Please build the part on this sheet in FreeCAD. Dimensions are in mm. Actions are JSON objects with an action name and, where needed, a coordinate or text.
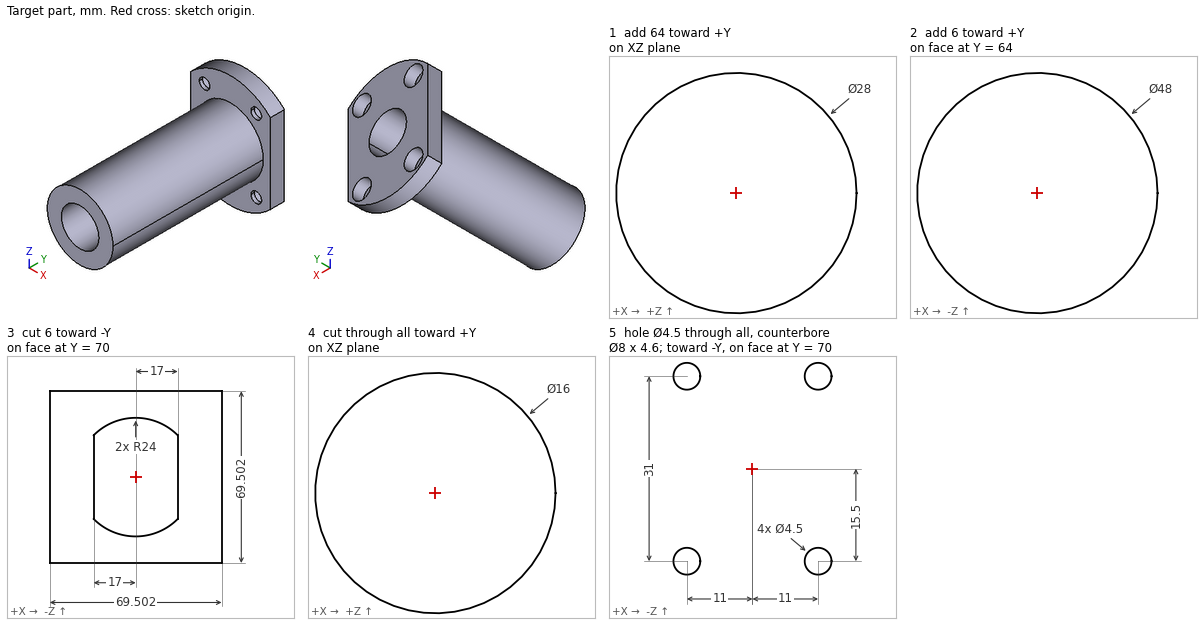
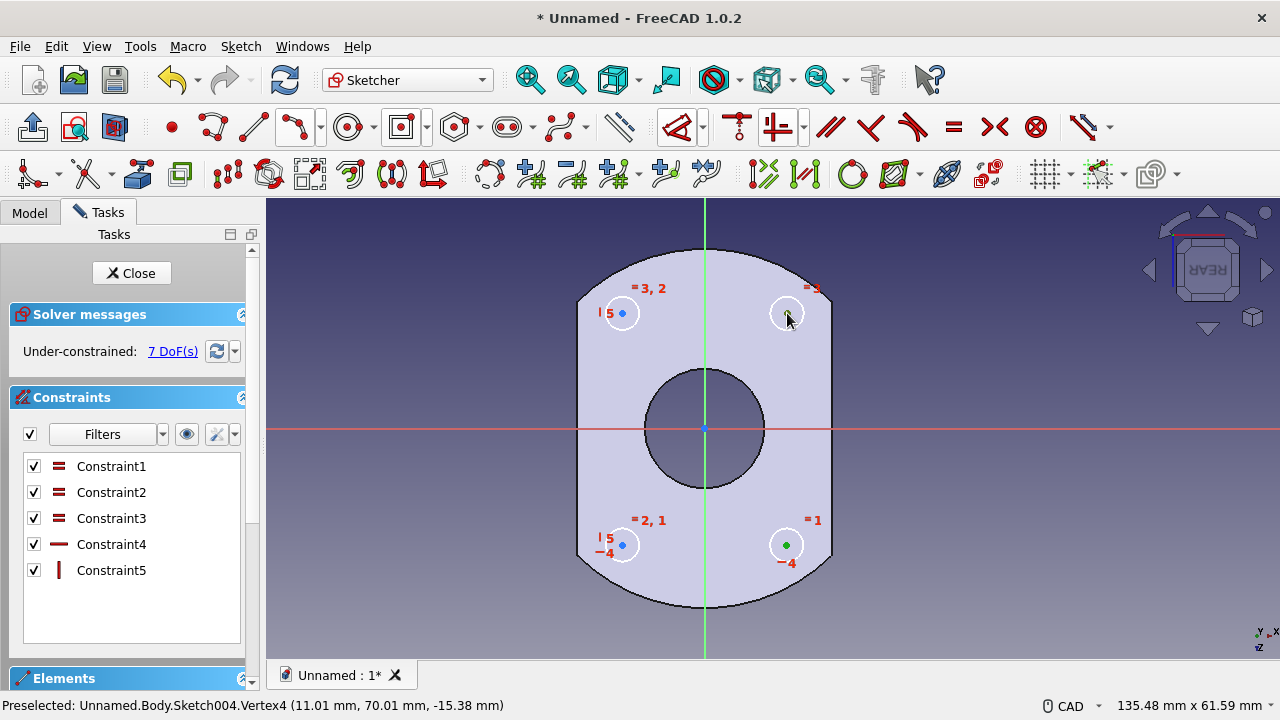
{"action": "key", "text": "v"}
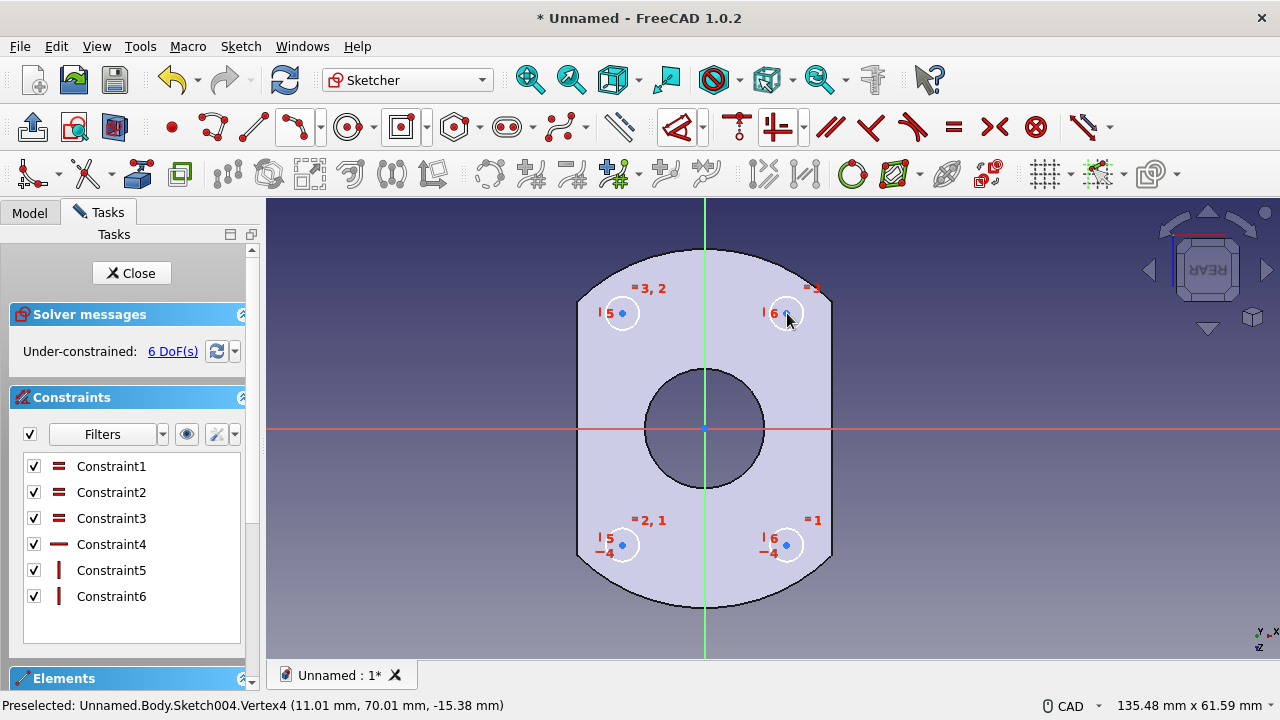
{"action": "left_click", "coordinate": [622, 313]}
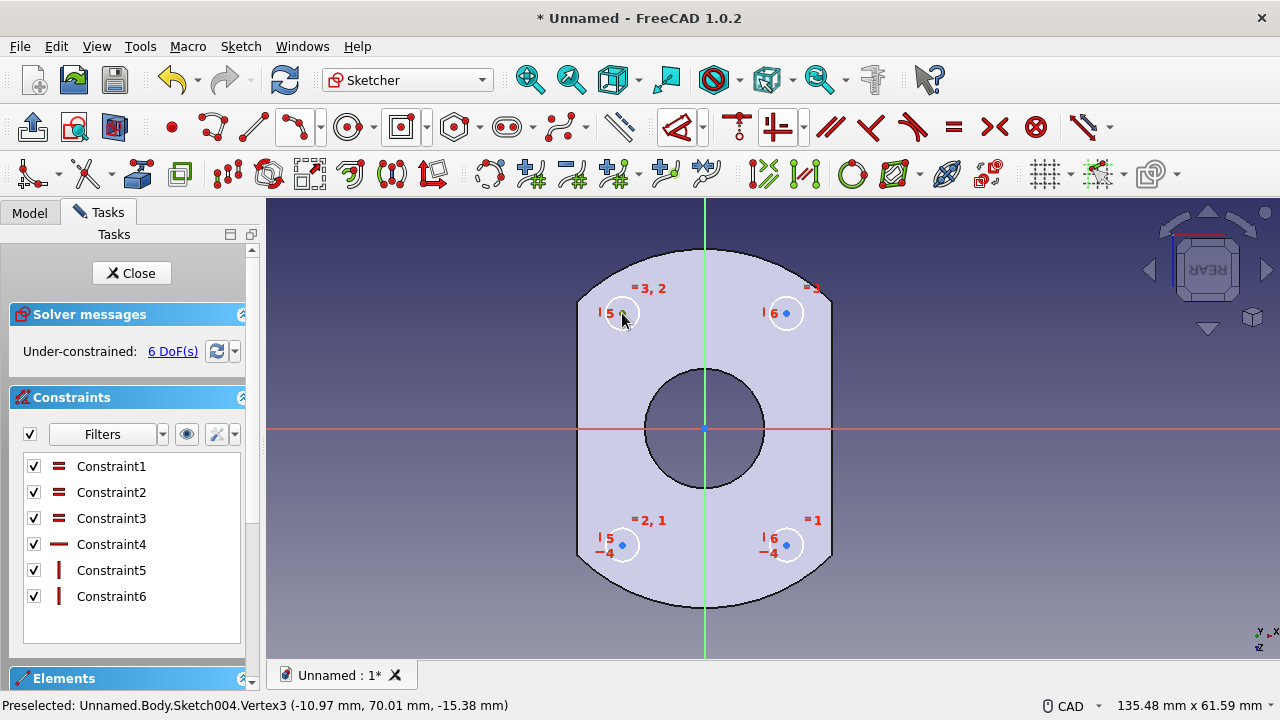
{"action": "left_click", "coordinate": [787, 313]}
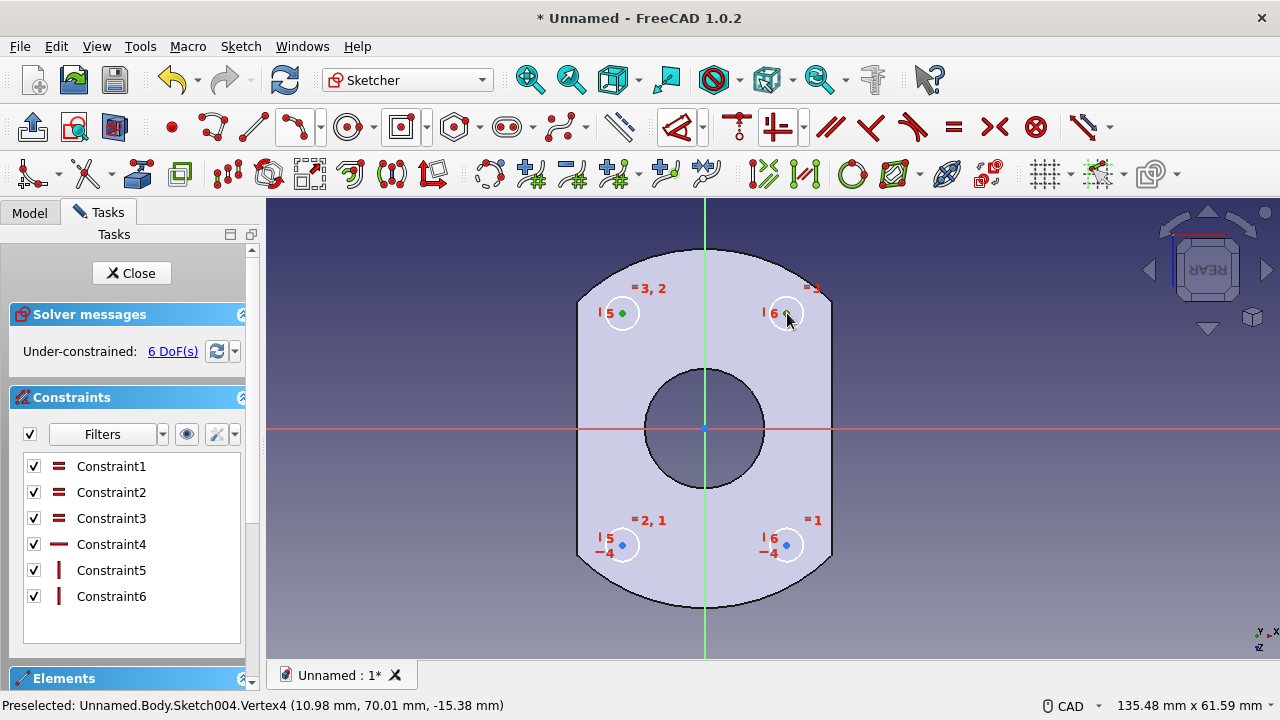
{"action": "left_click", "coordinate": [804, 128]}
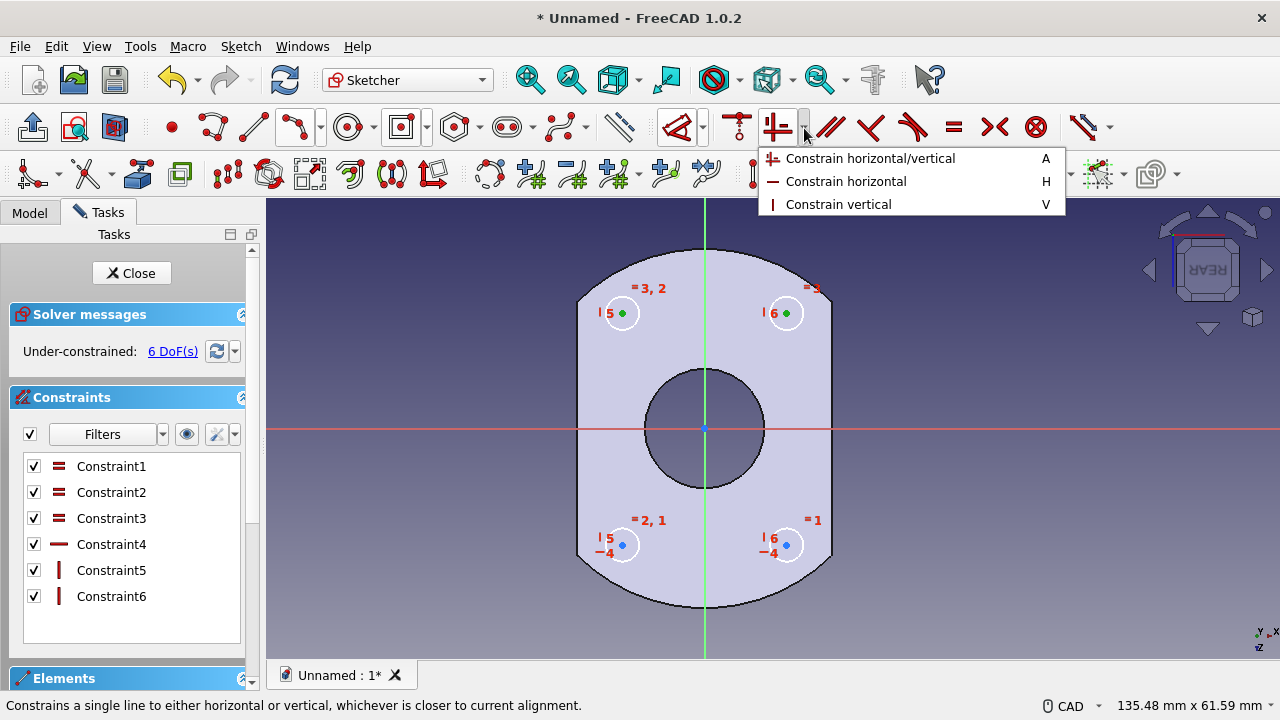
{"action": "left_click", "coordinate": [912, 182]}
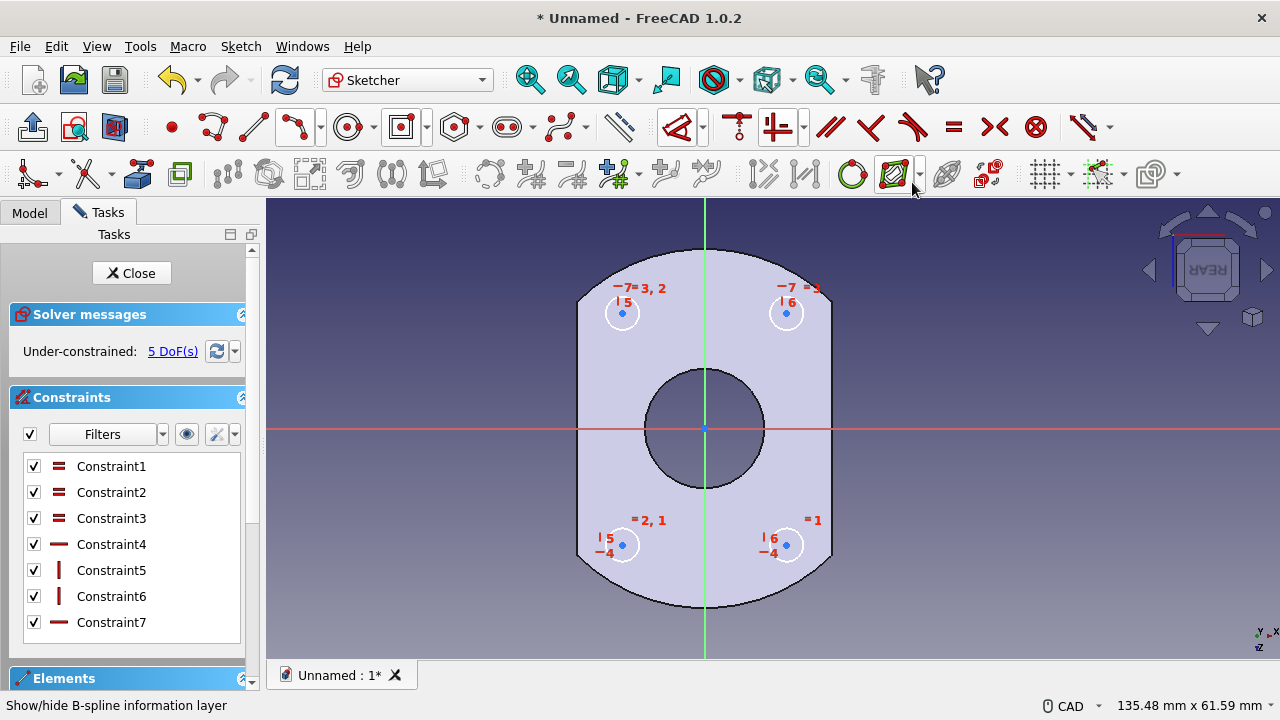
{"action": "left_click", "coordinate": [798, 533]}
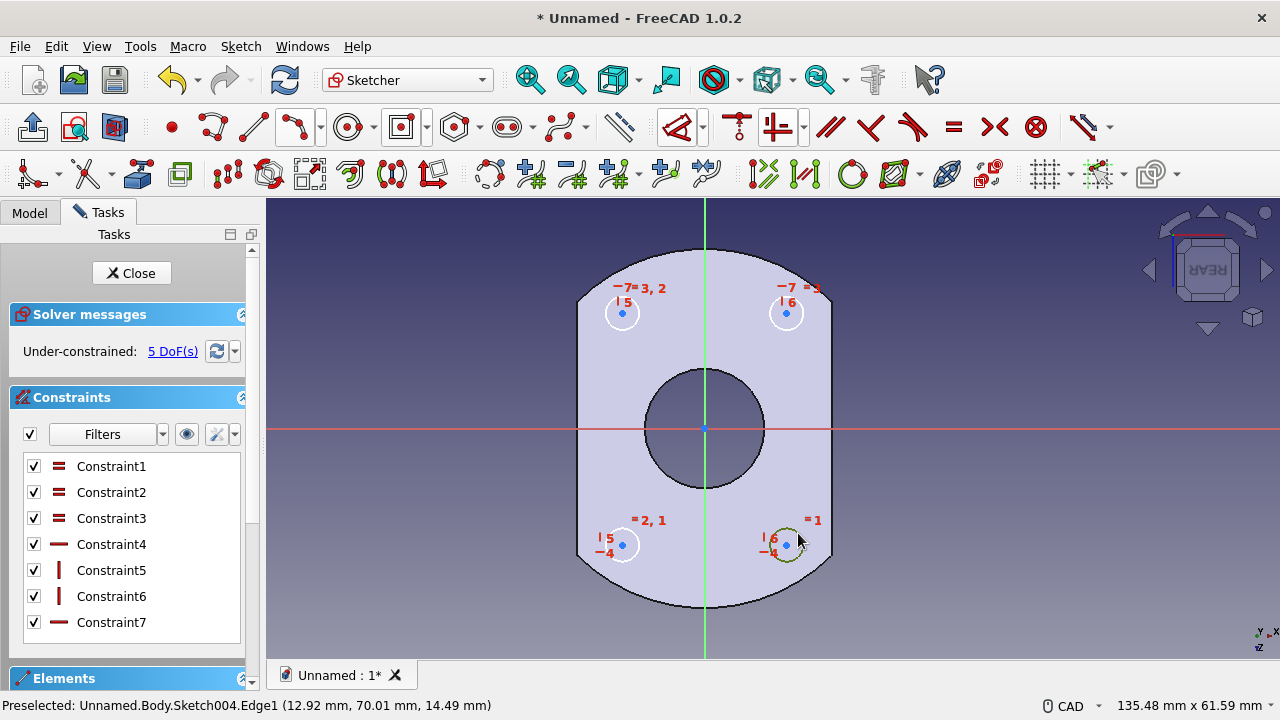
{"action": "left_click", "coordinate": [702, 128]}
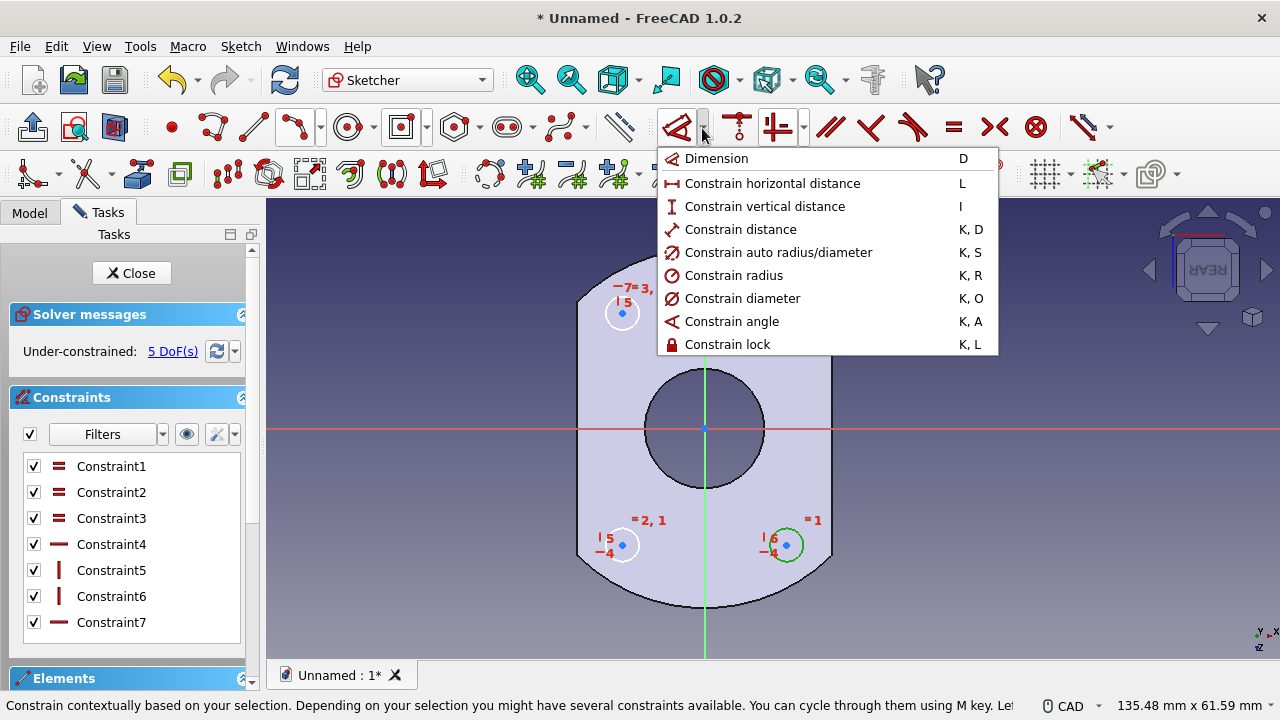
{"action": "left_click", "coordinate": [828, 298]}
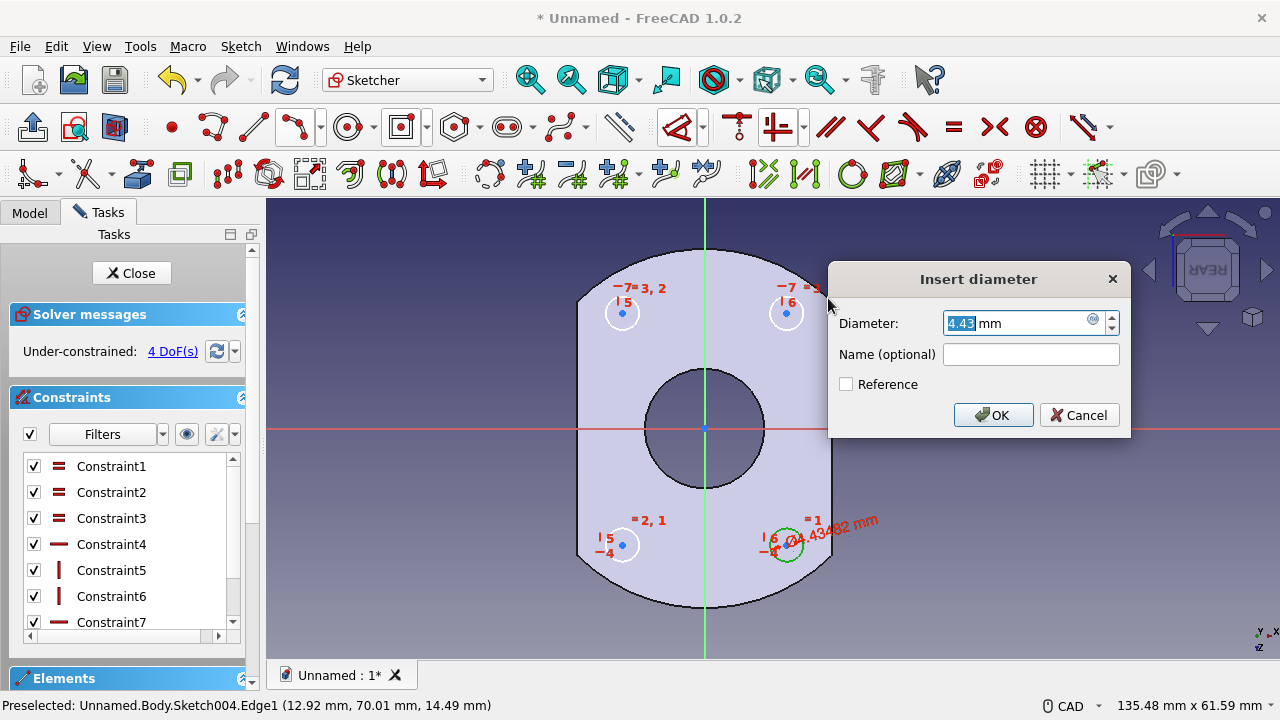
{"action": "type", "text": "4.5"}
{"action": "key", "text": "Return"}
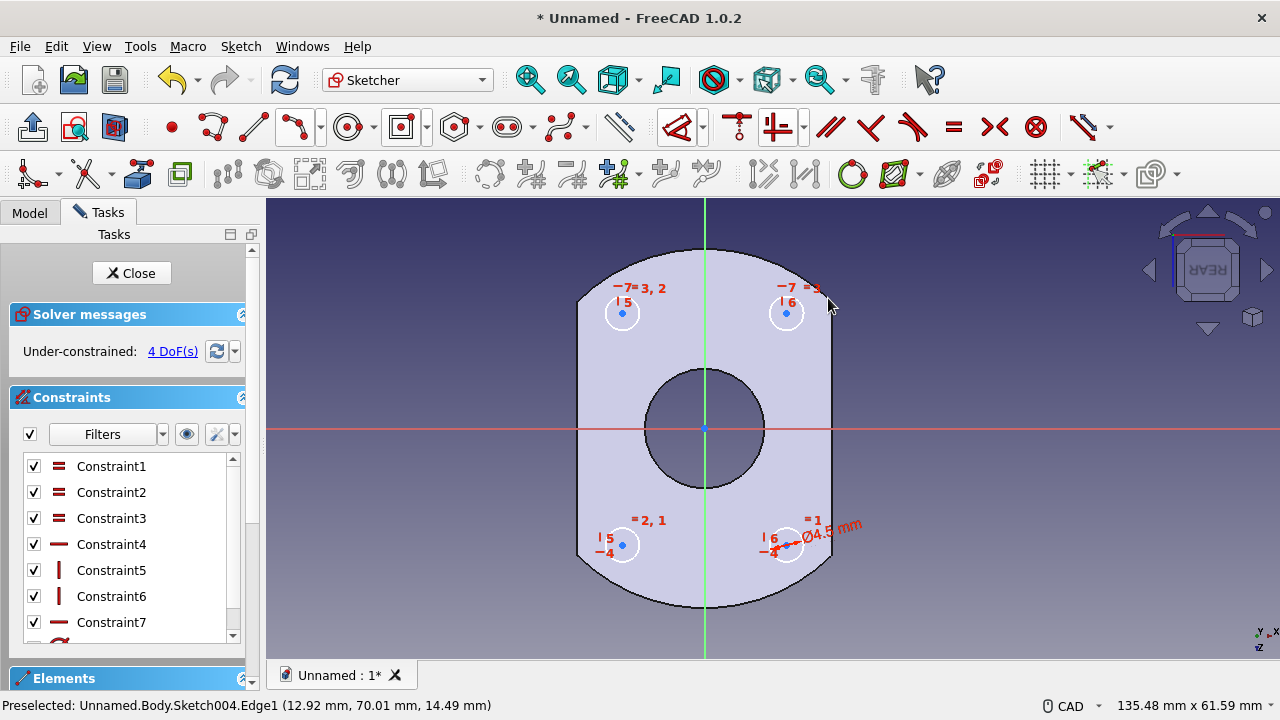
{"action": "left_click", "coordinate": [787, 545]}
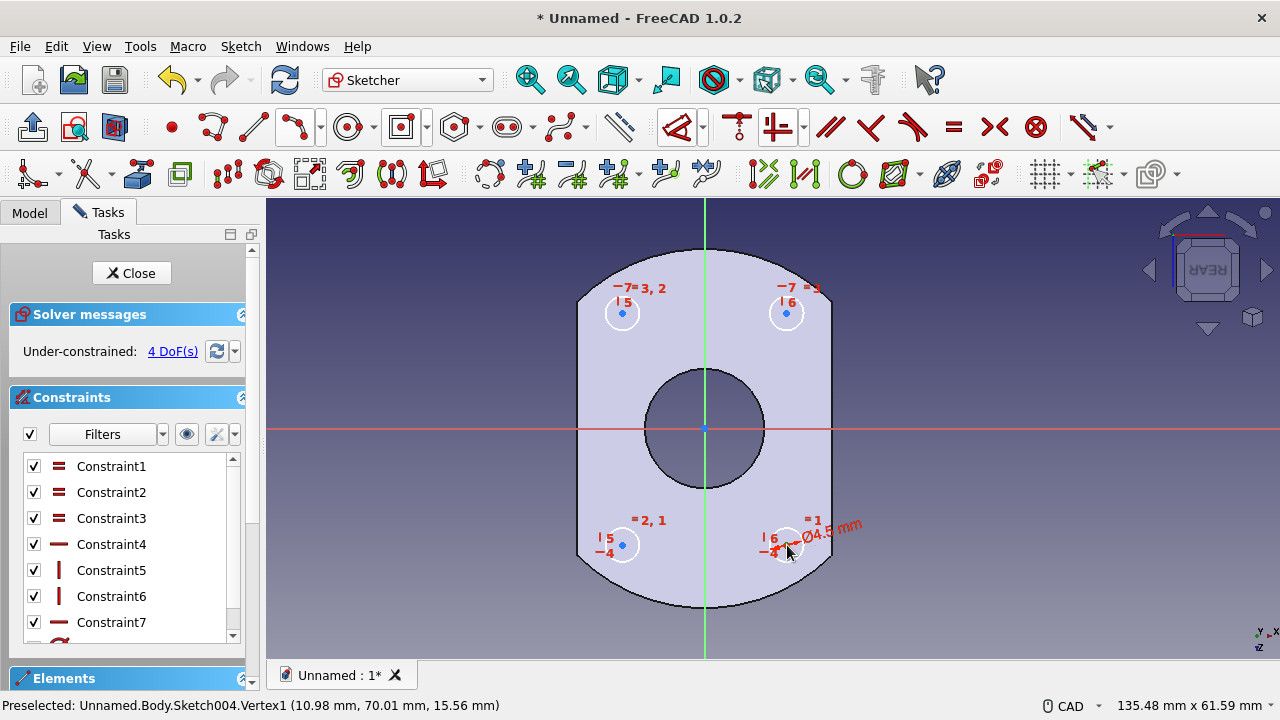
{"action": "key", "text": "l"}